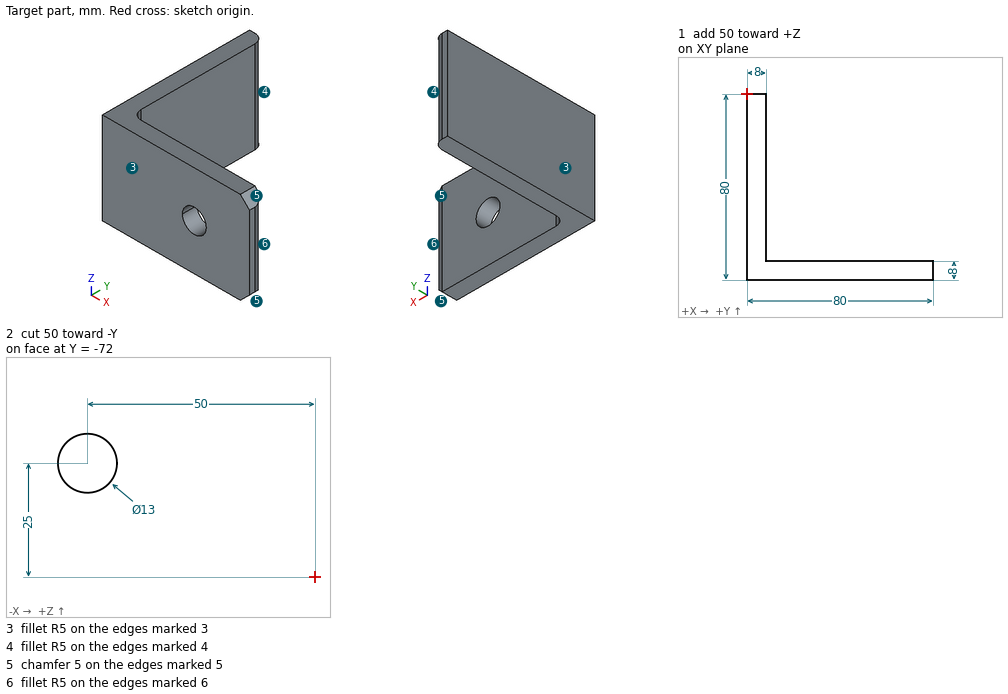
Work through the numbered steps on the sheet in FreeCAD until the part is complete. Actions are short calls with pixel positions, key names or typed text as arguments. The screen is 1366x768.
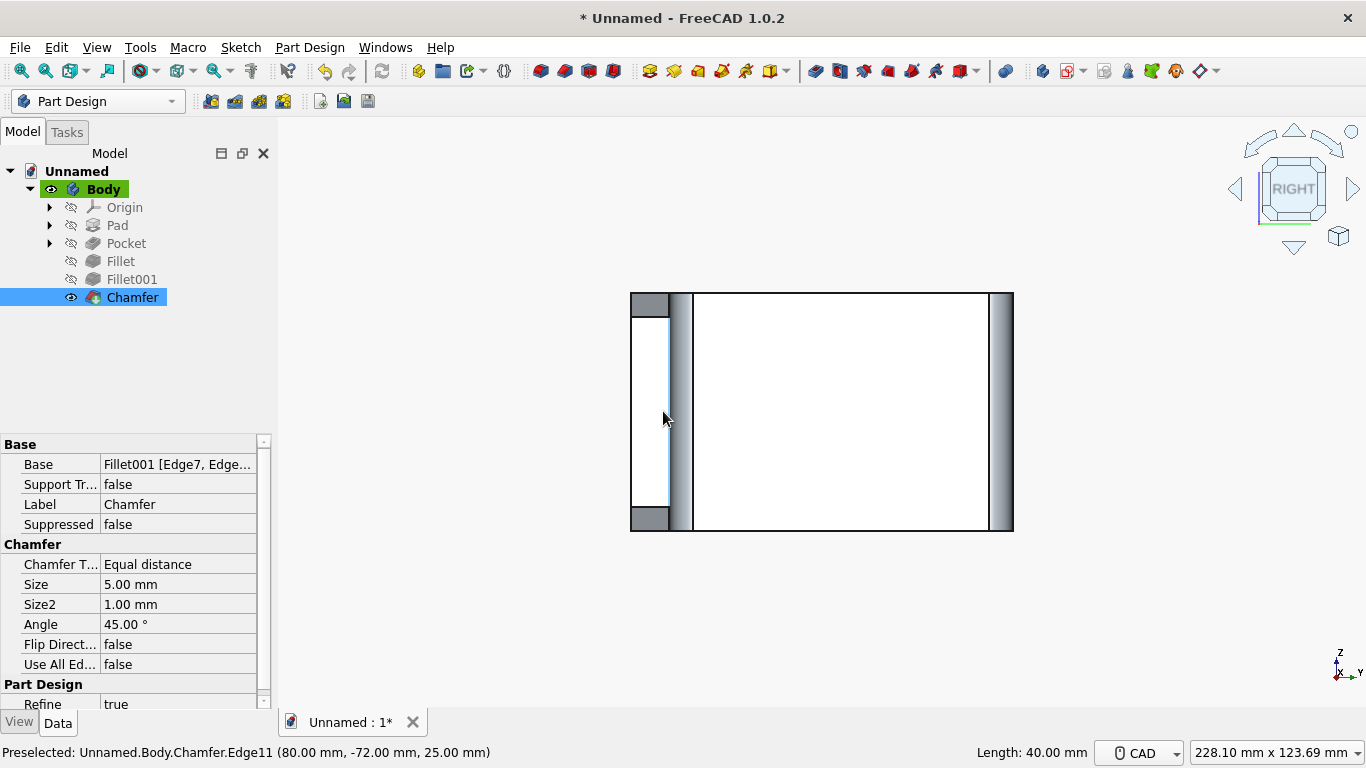
click(542, 72)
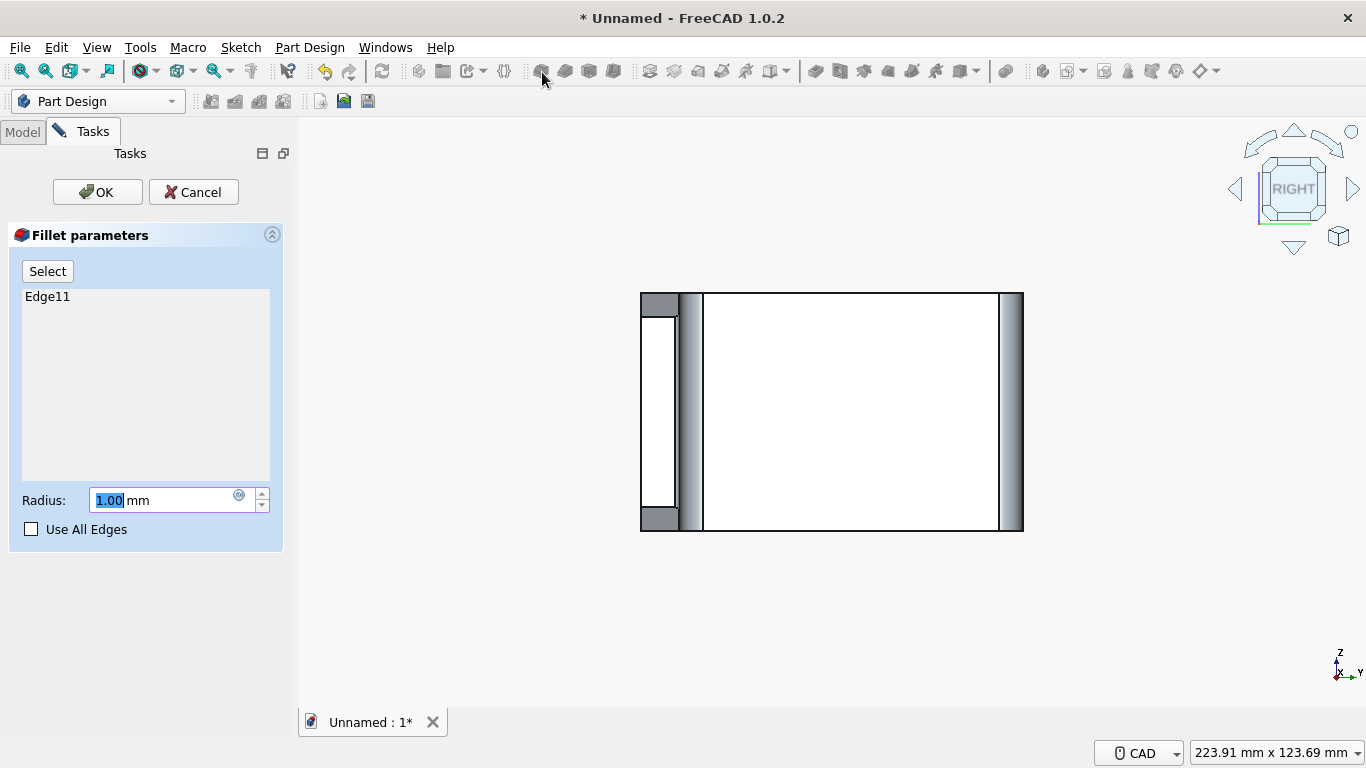
text(5)
key(Tab)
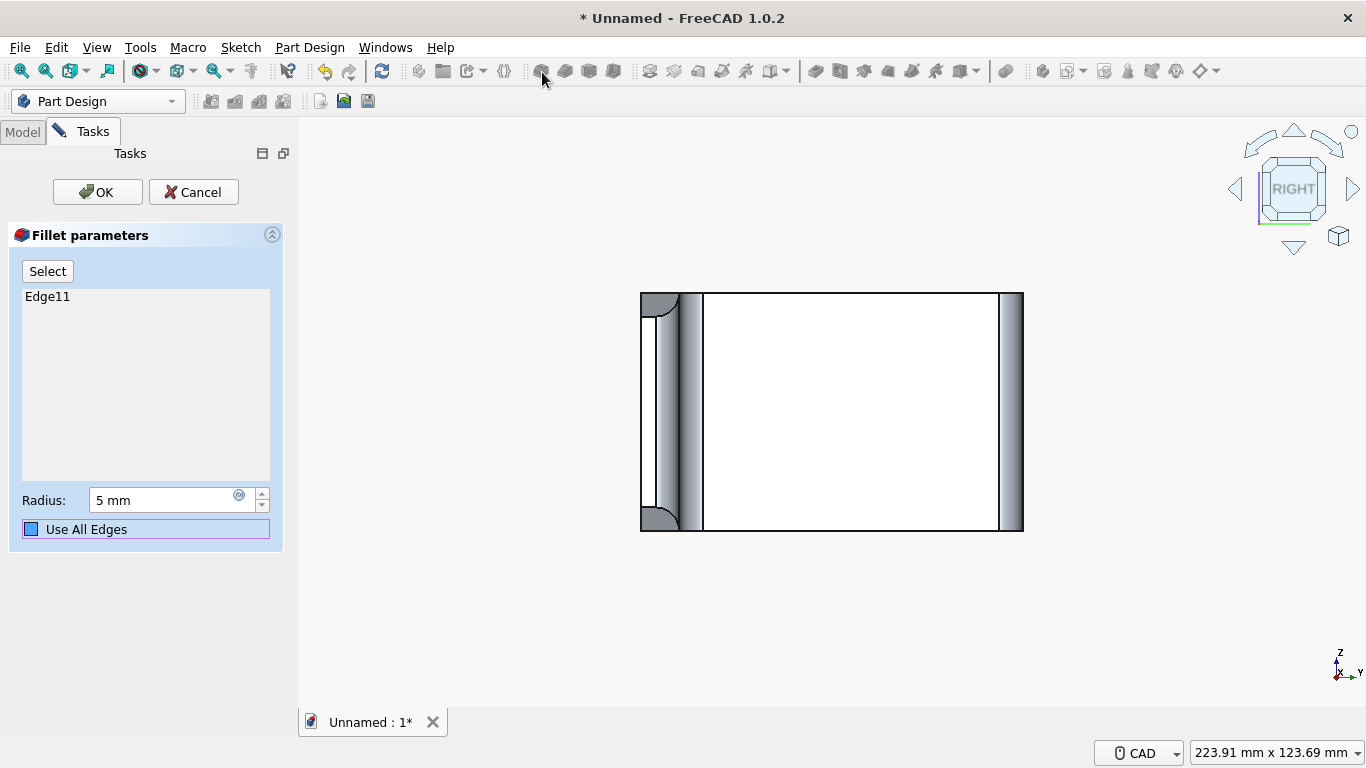
click(98, 192)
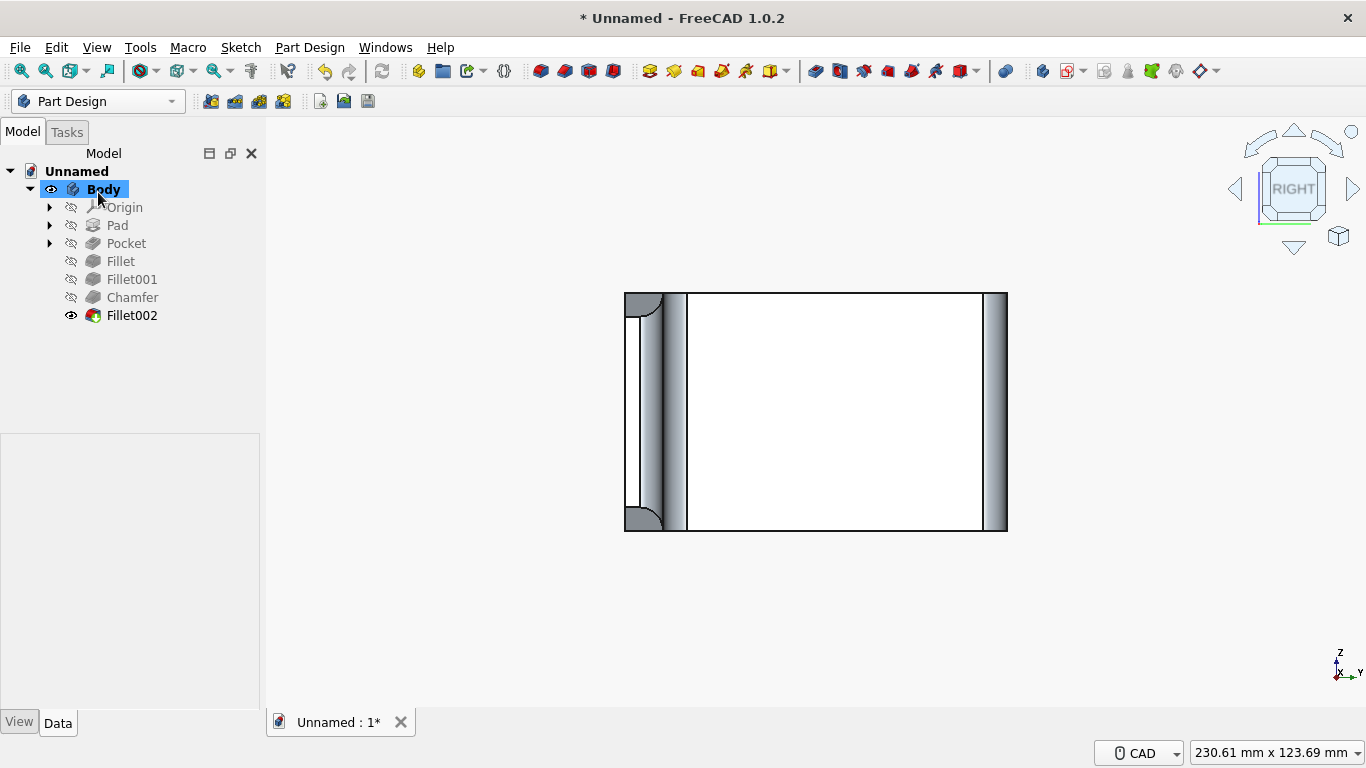
key(0)